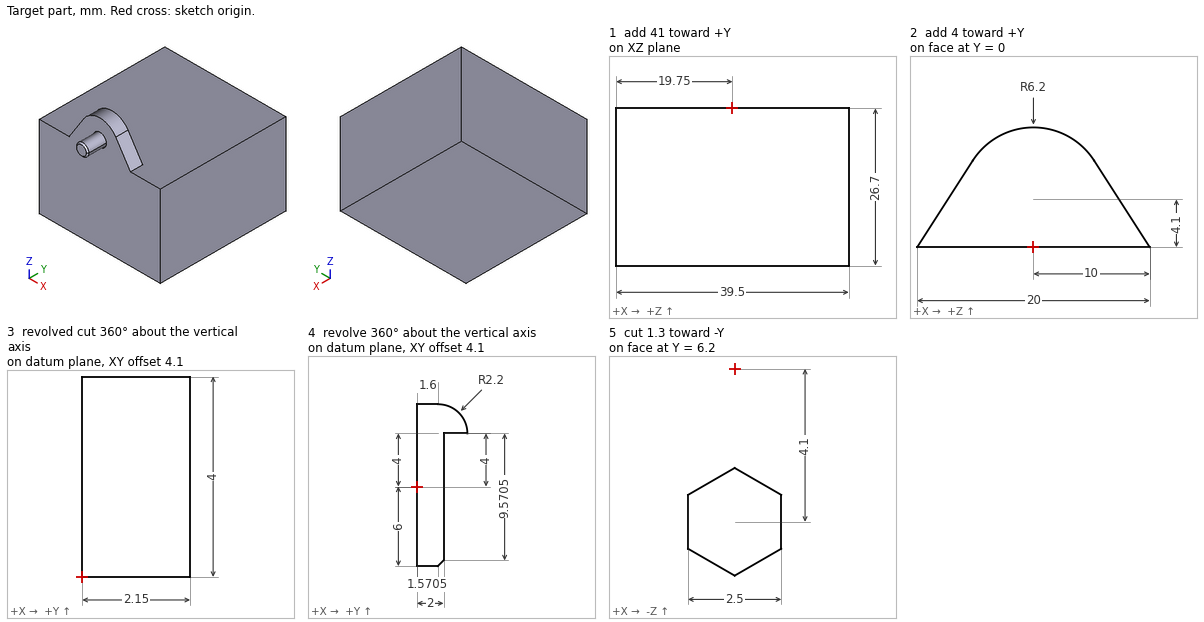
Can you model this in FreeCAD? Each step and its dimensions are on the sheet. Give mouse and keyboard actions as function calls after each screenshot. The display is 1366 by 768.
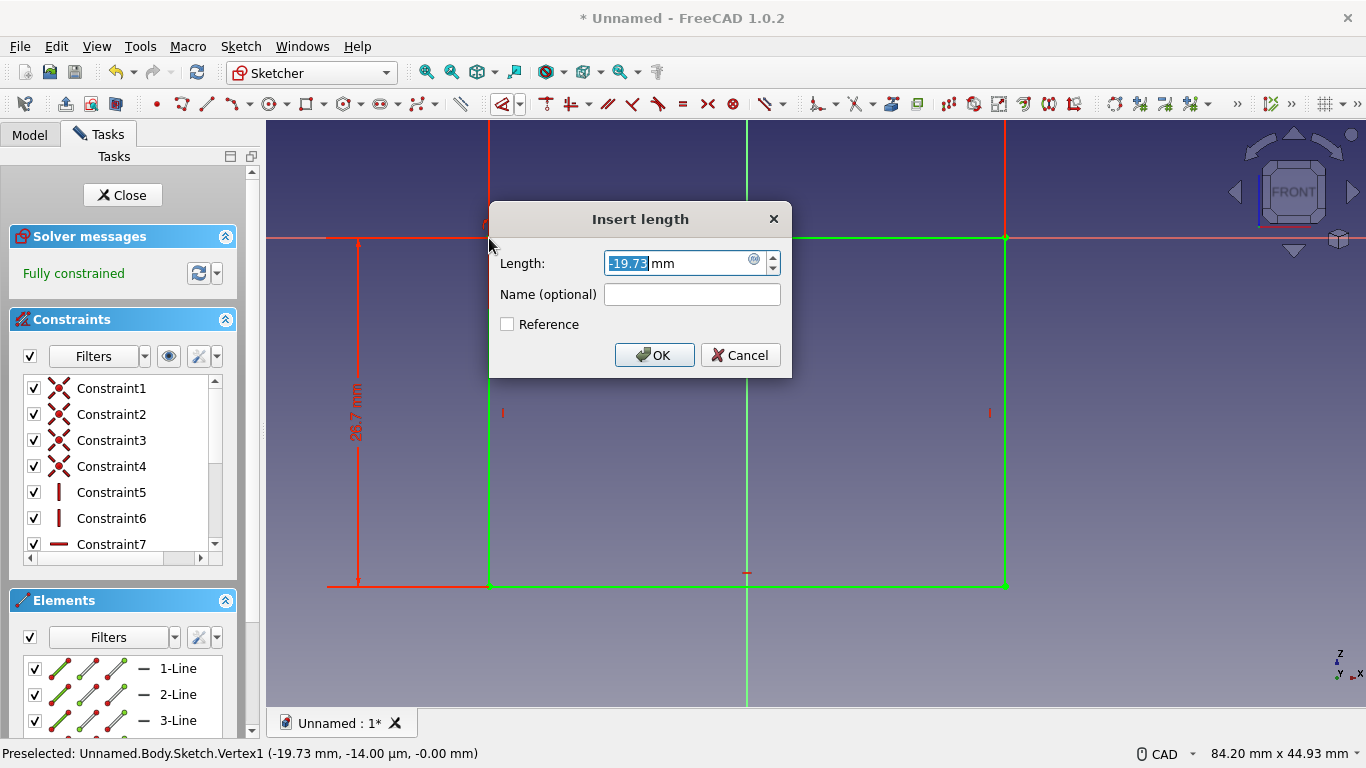
text(-19.75)
key(Return)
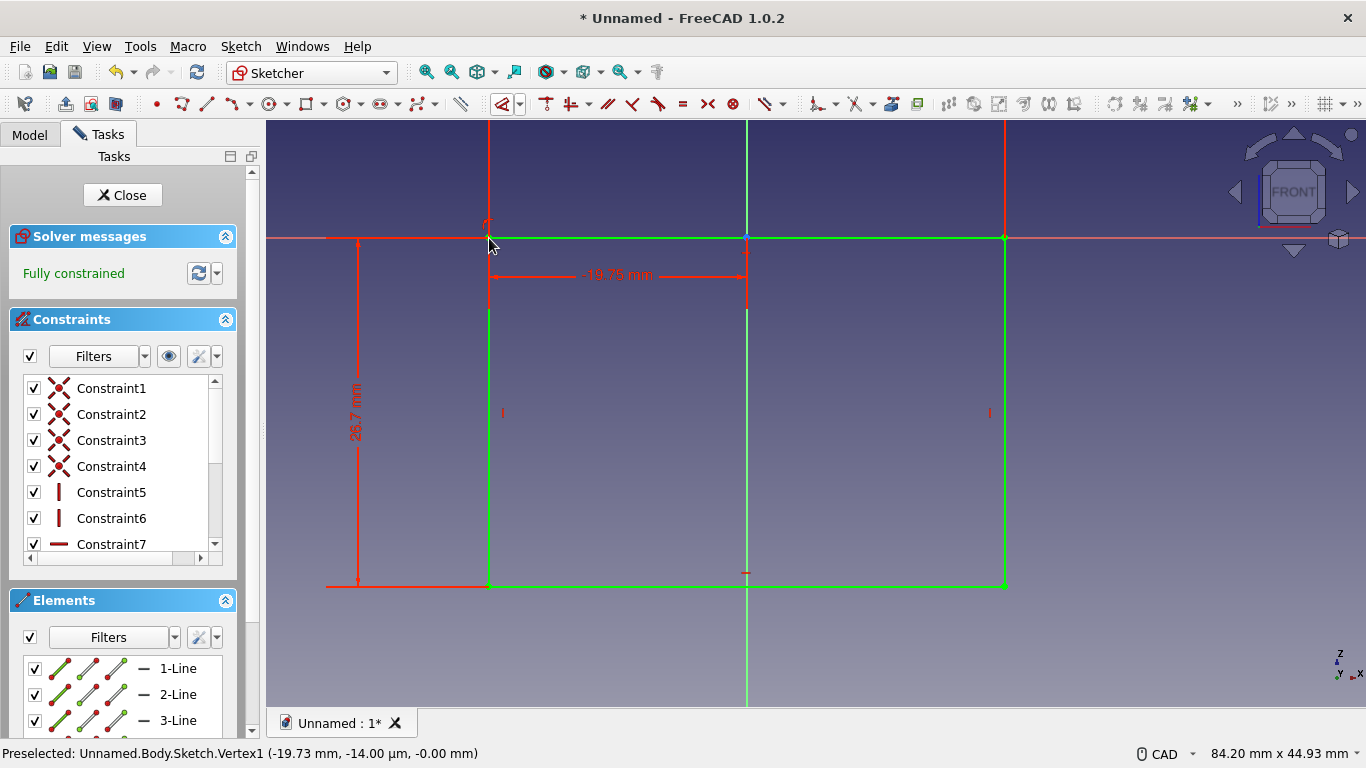
click(123, 195)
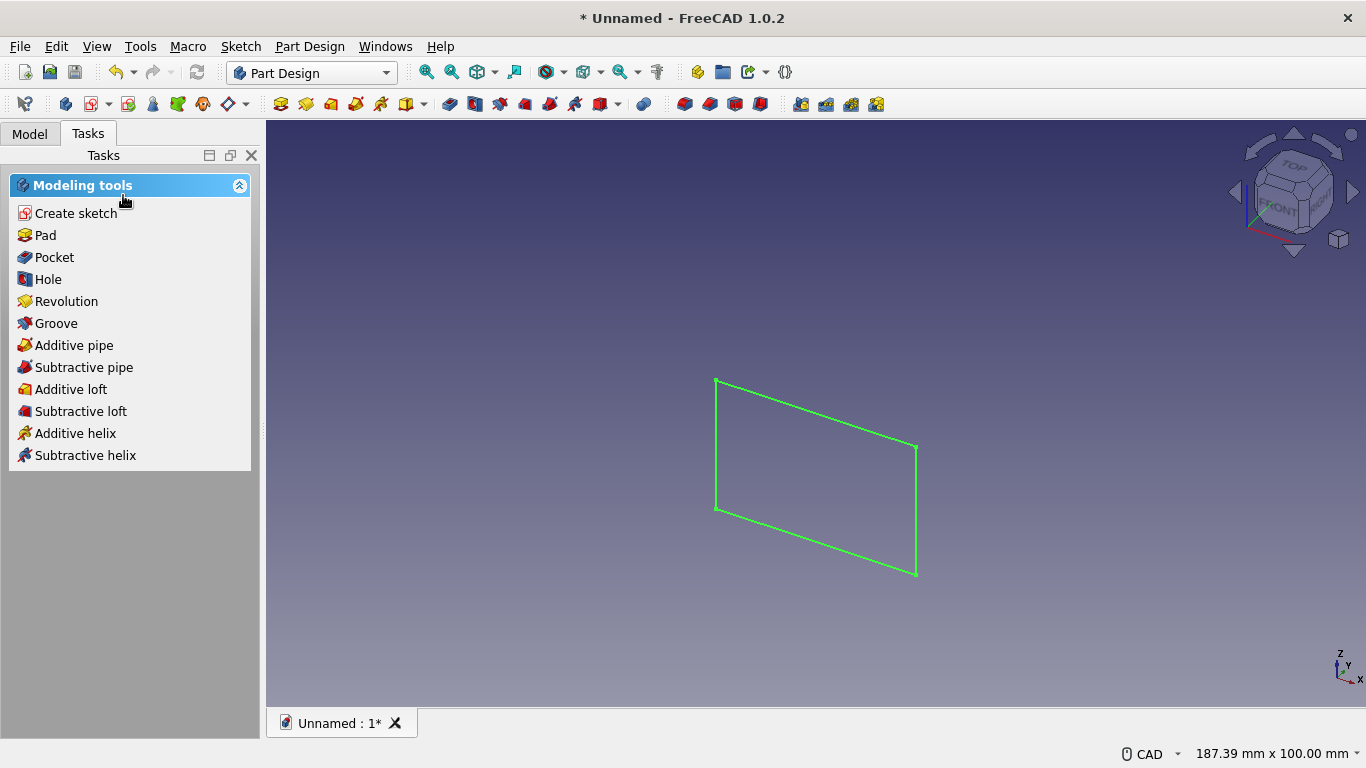
click(281, 104)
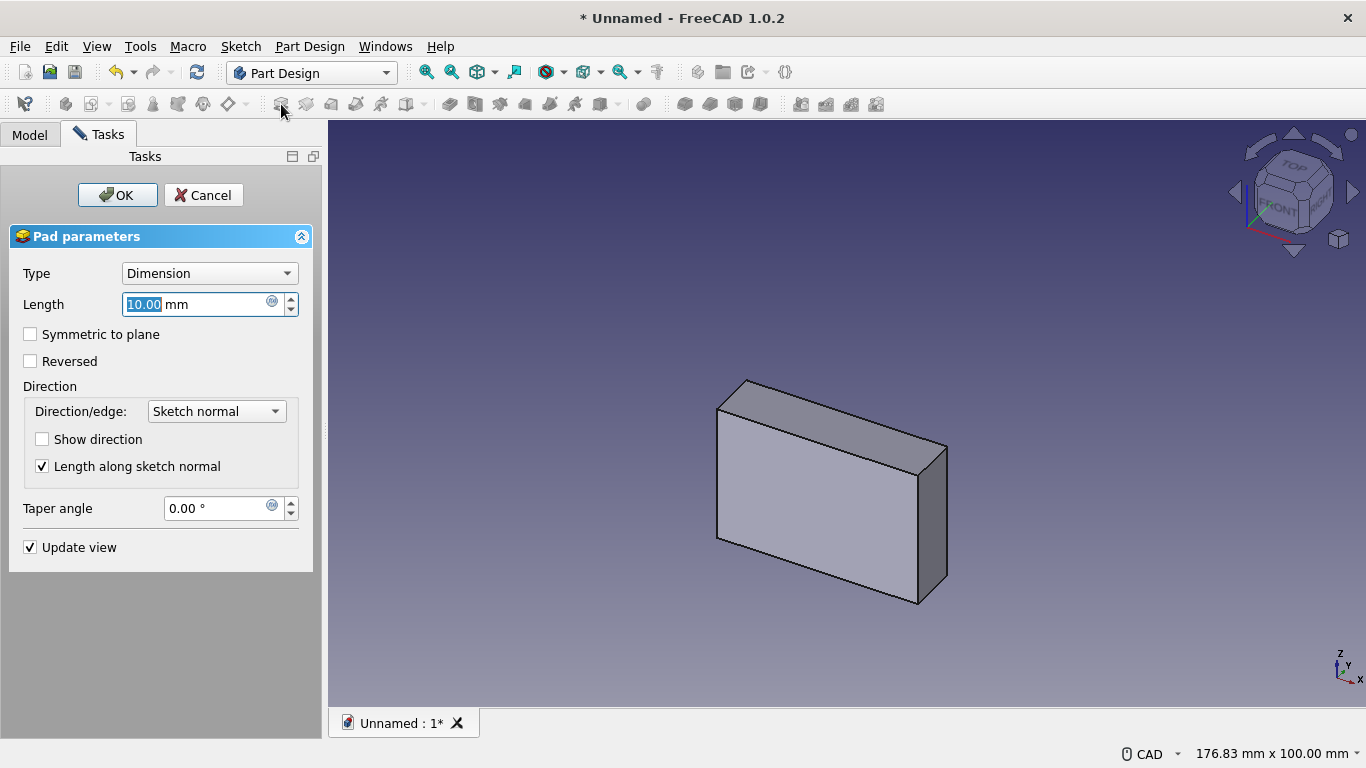
text(41)
key(Tab)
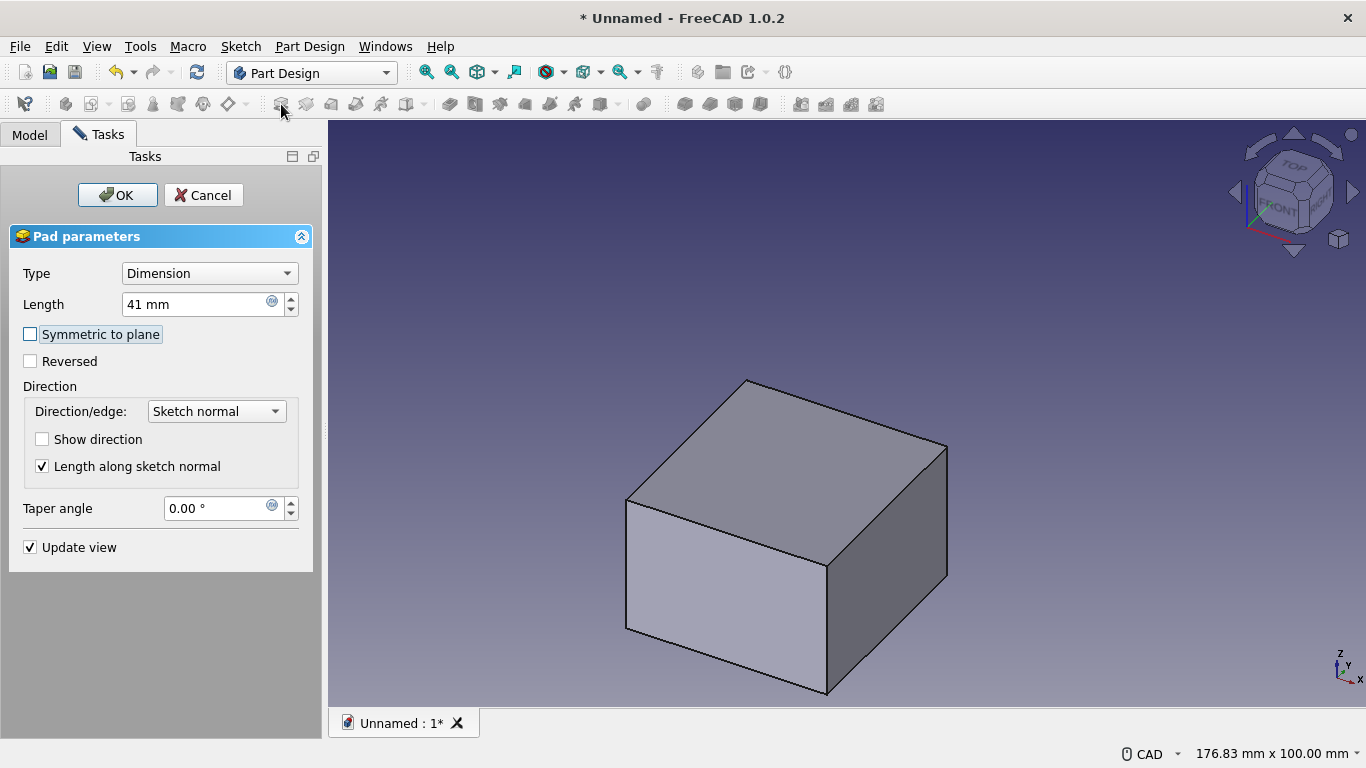
click(31, 361)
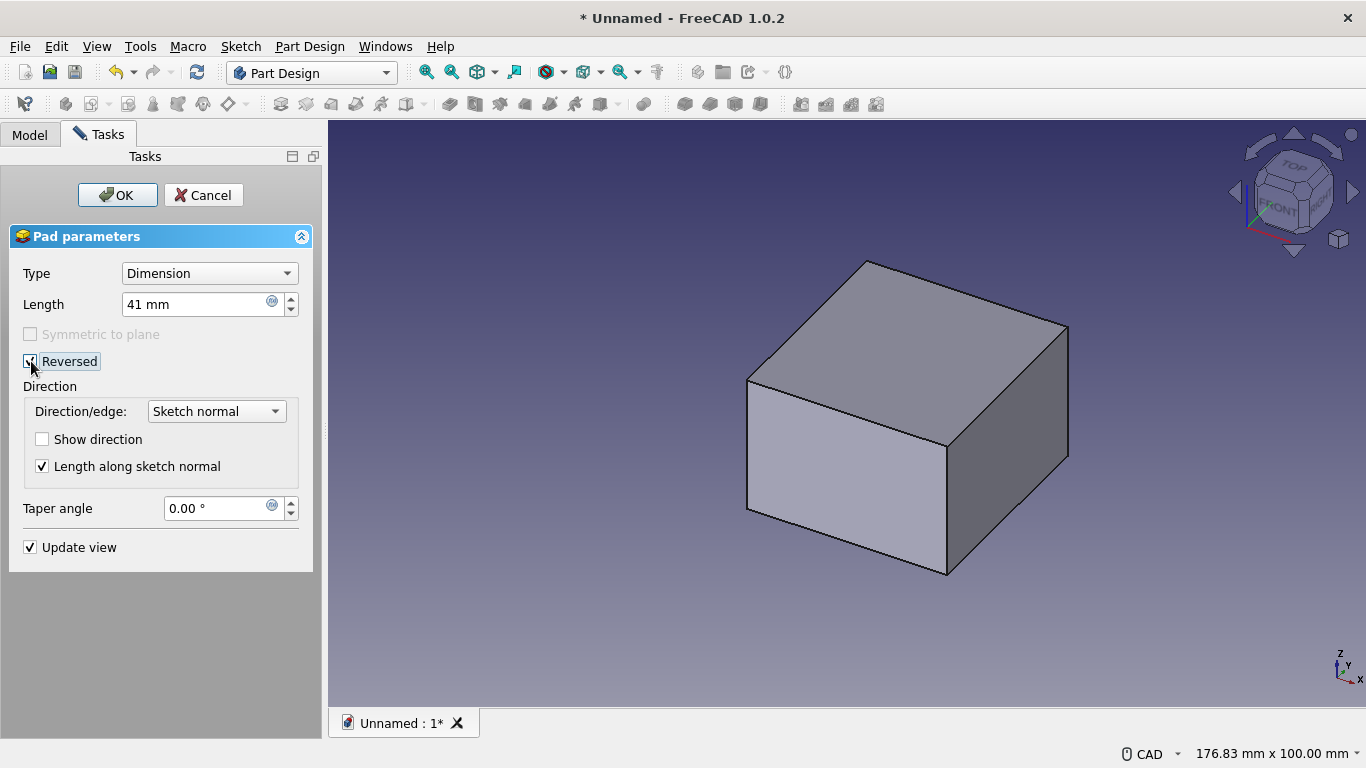
click(118, 195)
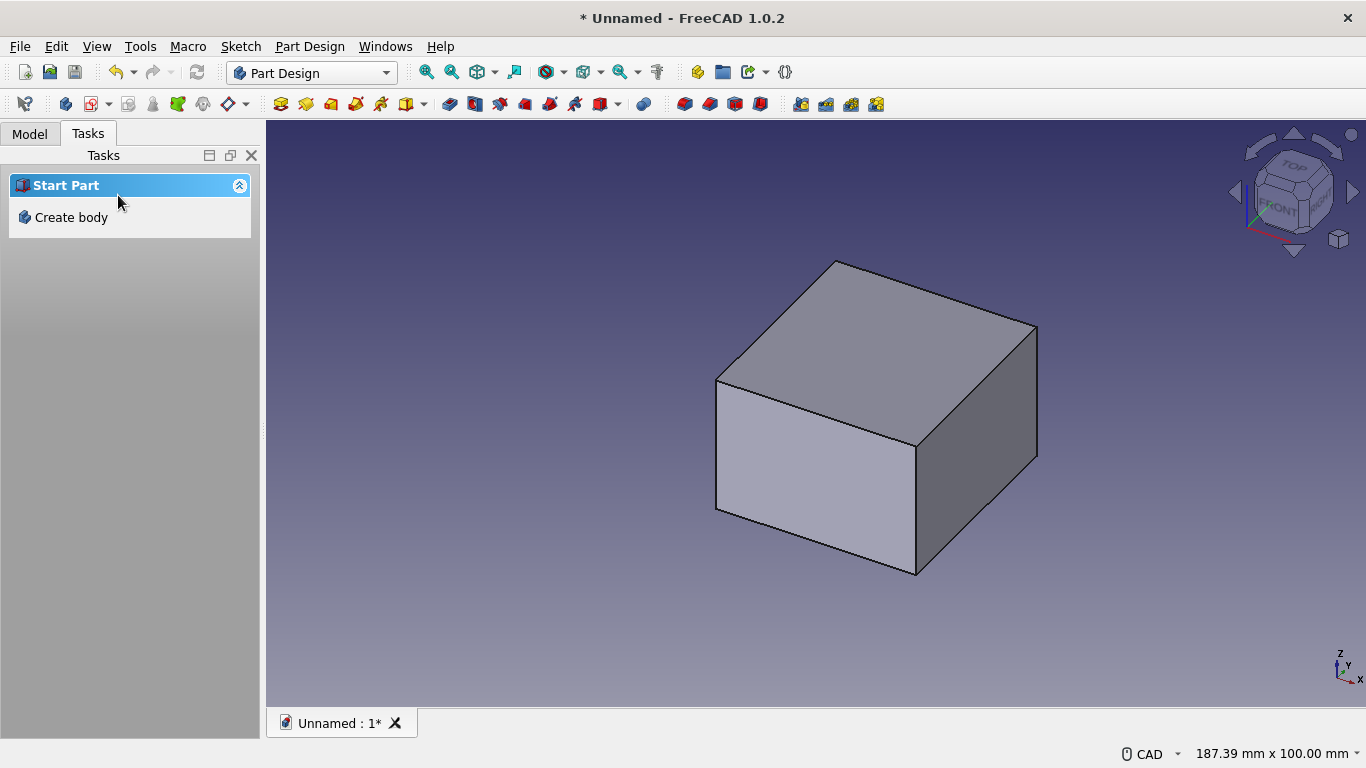
click(845, 486)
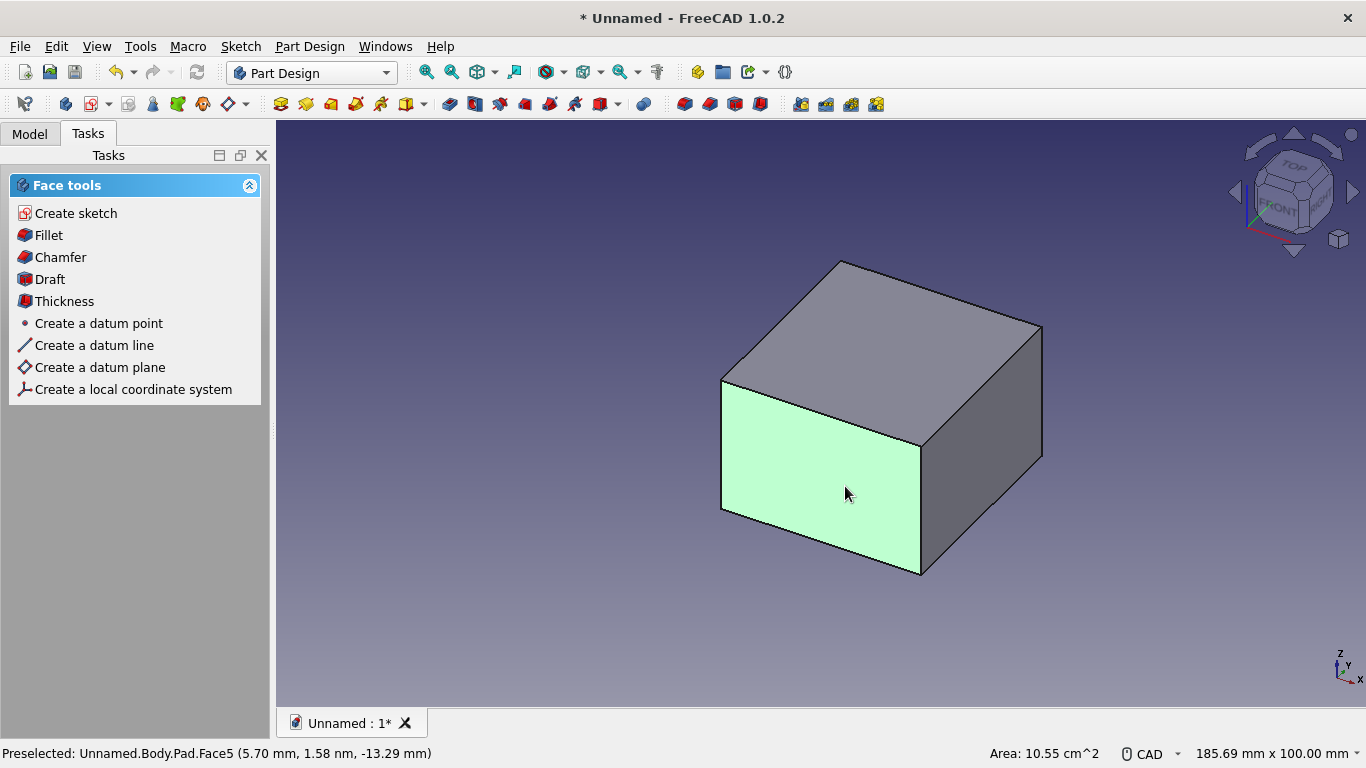
click(90, 104)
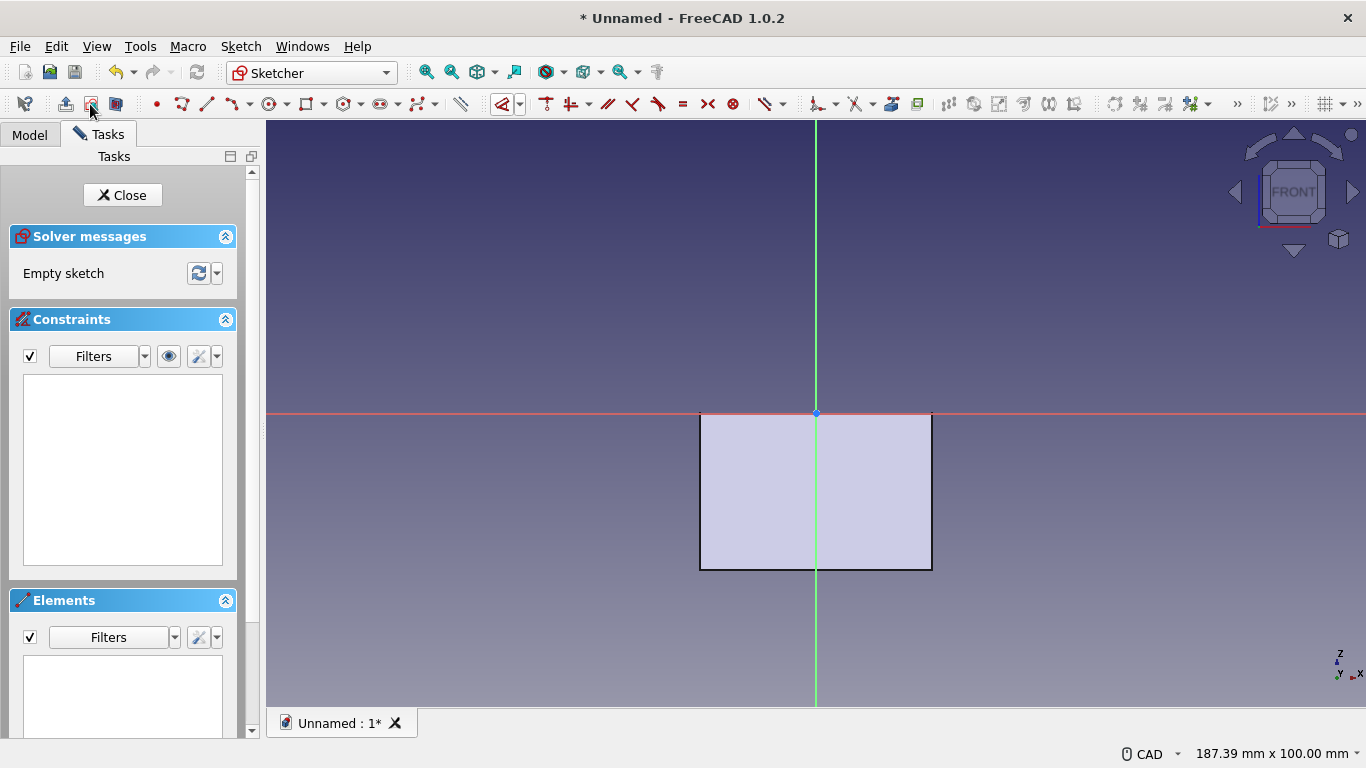
scroll(833, 376, up, 8)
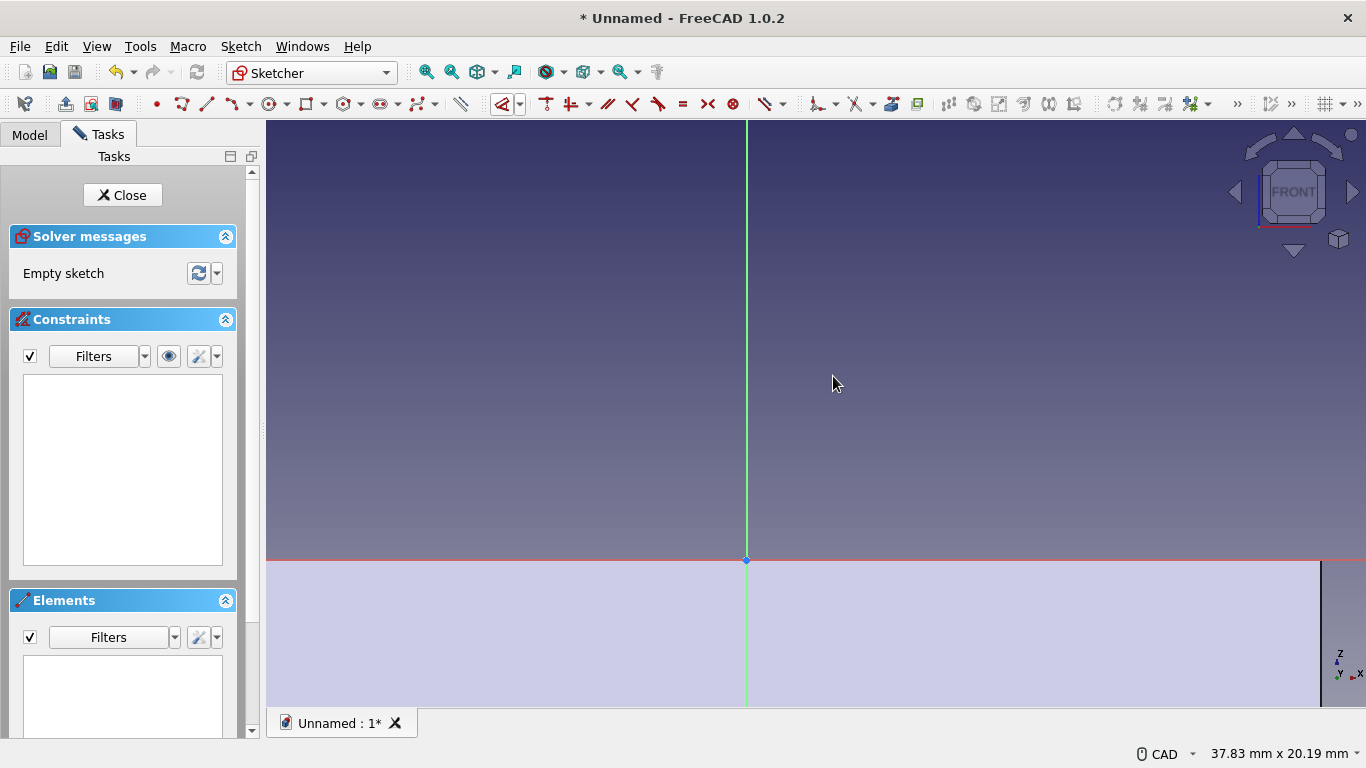
key(g)
key(m)